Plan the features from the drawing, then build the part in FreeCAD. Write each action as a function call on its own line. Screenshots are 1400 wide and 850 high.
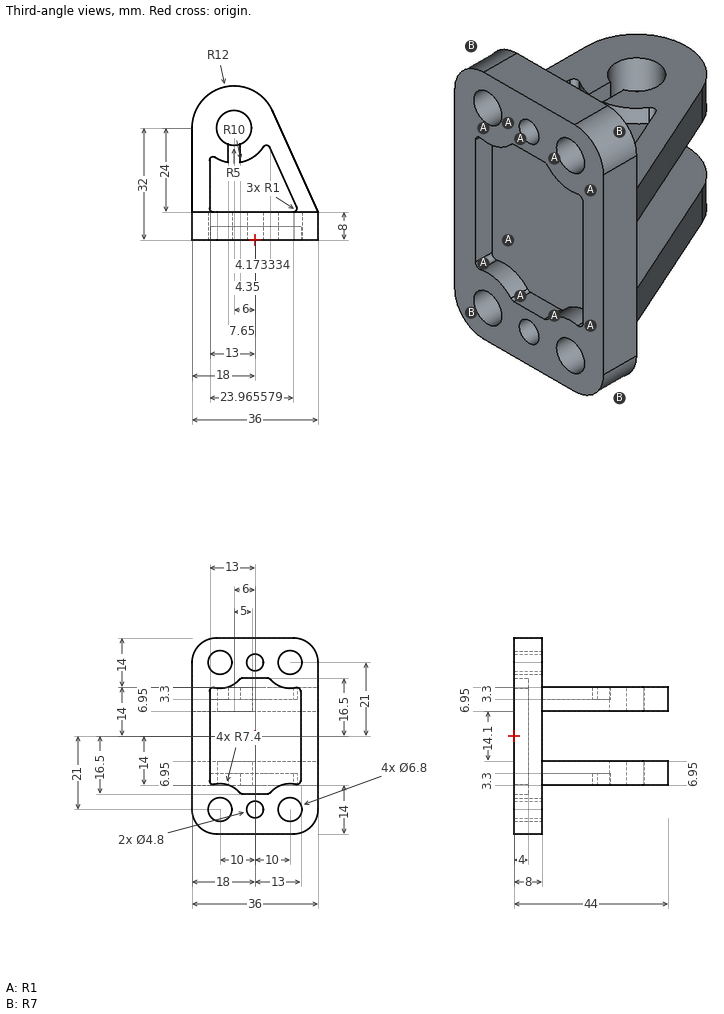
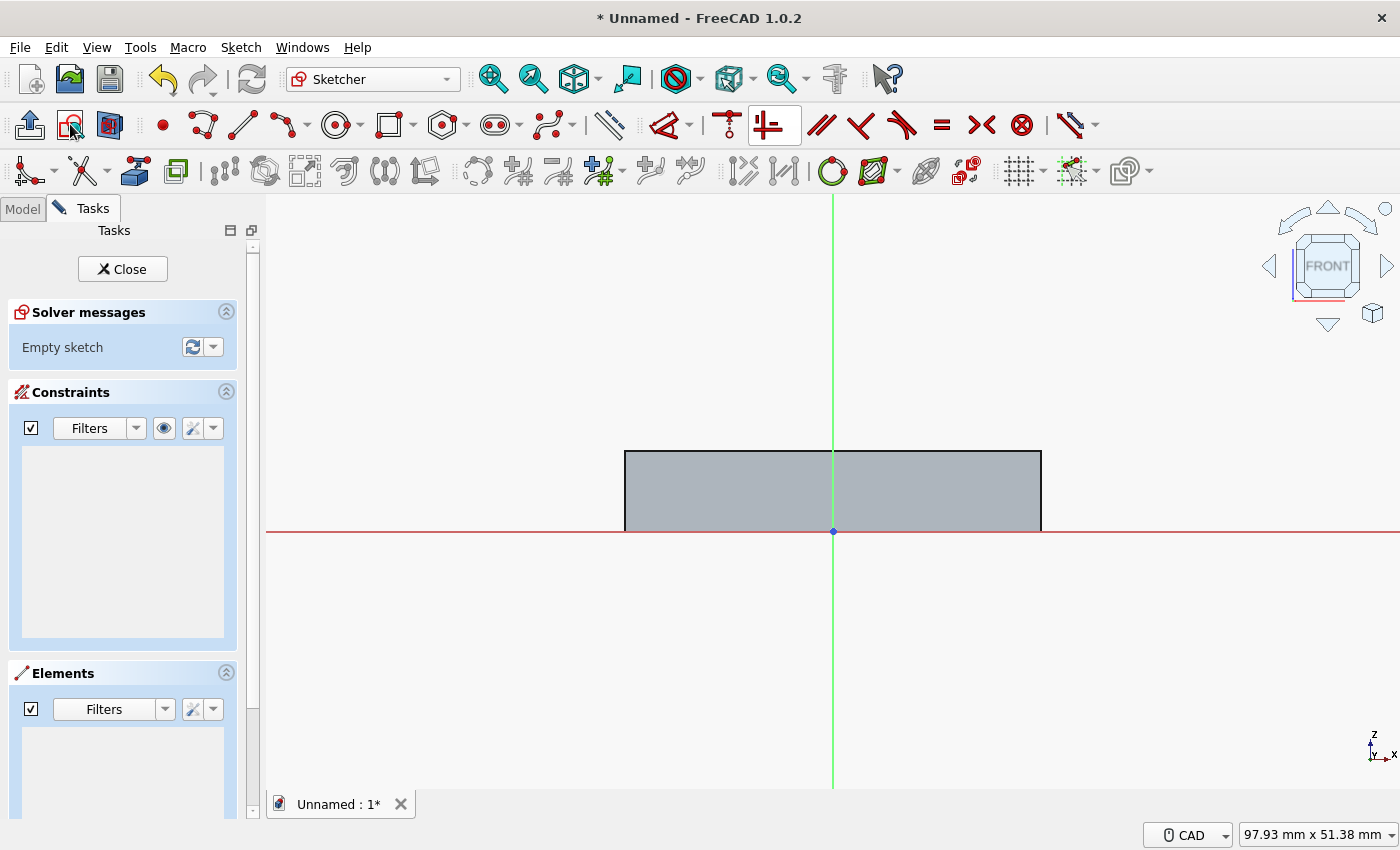
scroll(972, 492, up, 2)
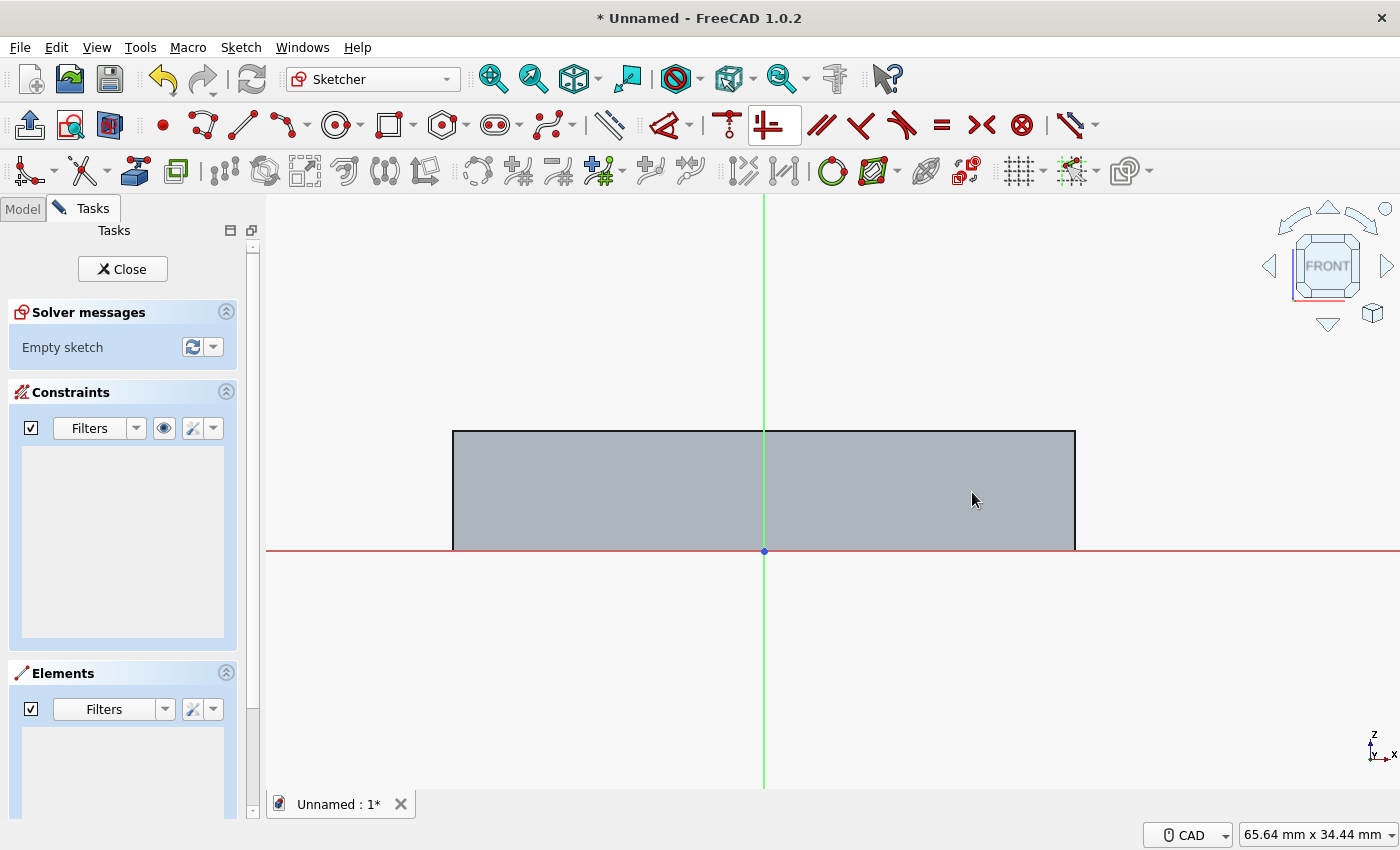
key(g)
key(r)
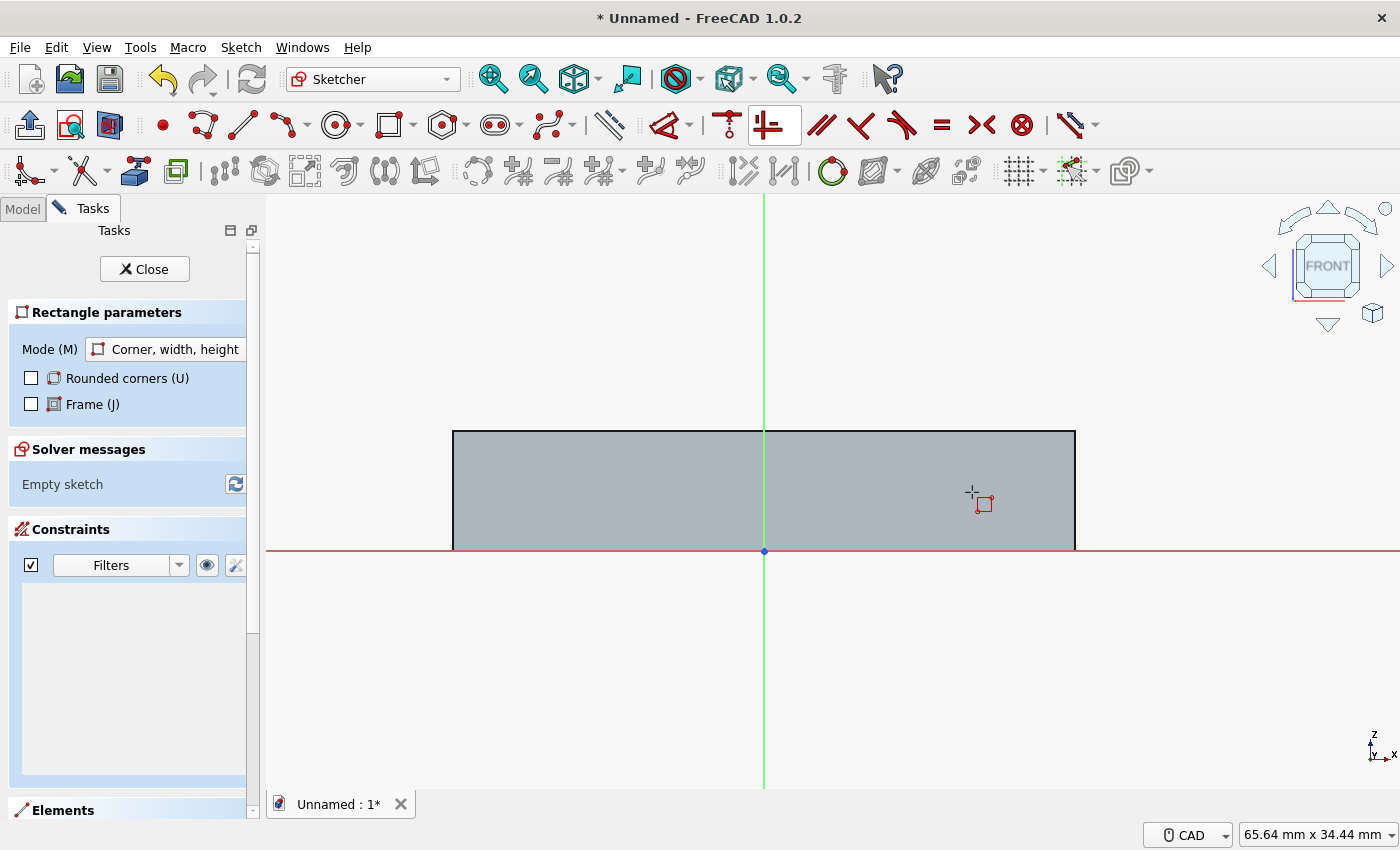
click(453, 431)
click(1075, 551)
key(Escape)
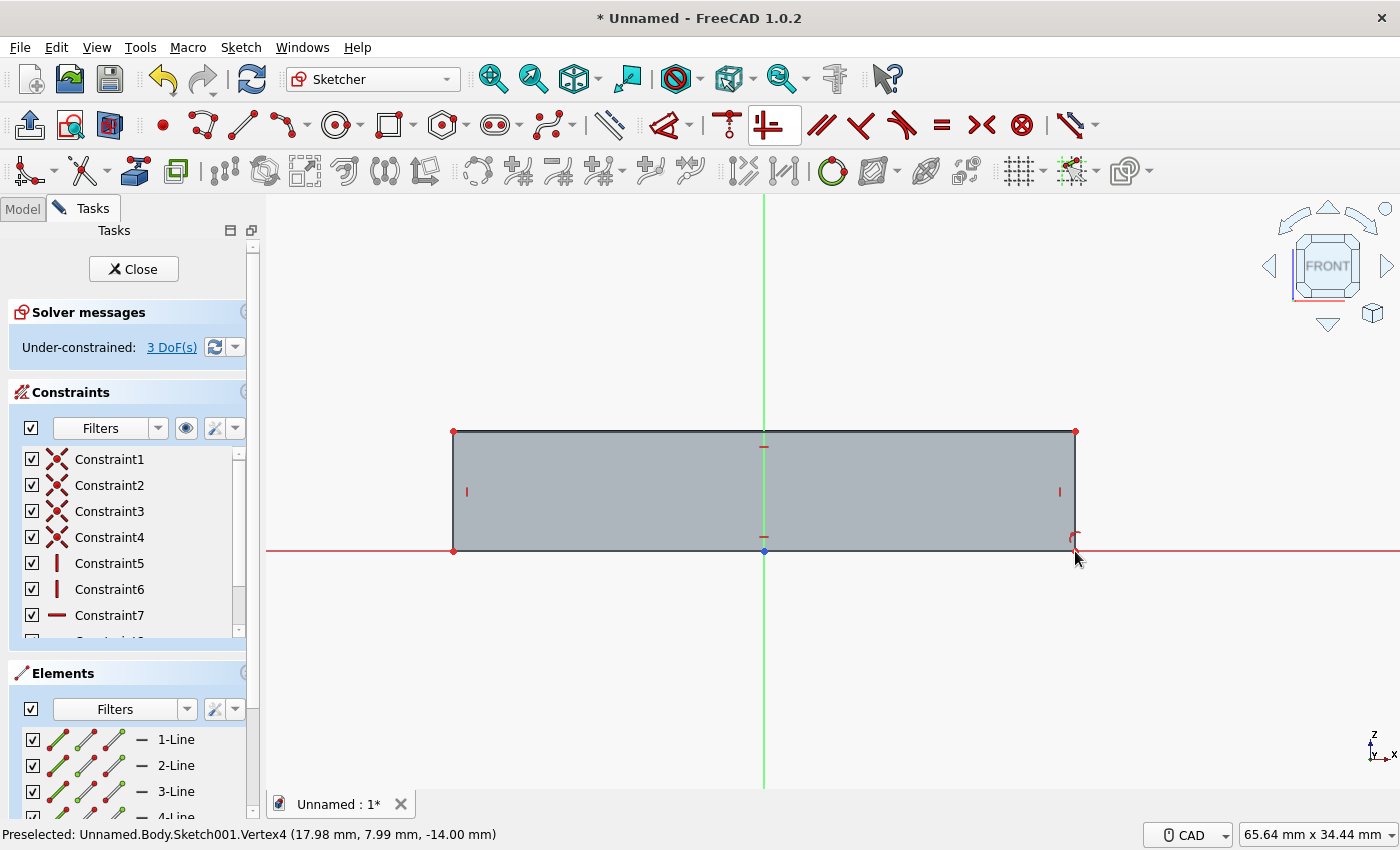
click(640, 551)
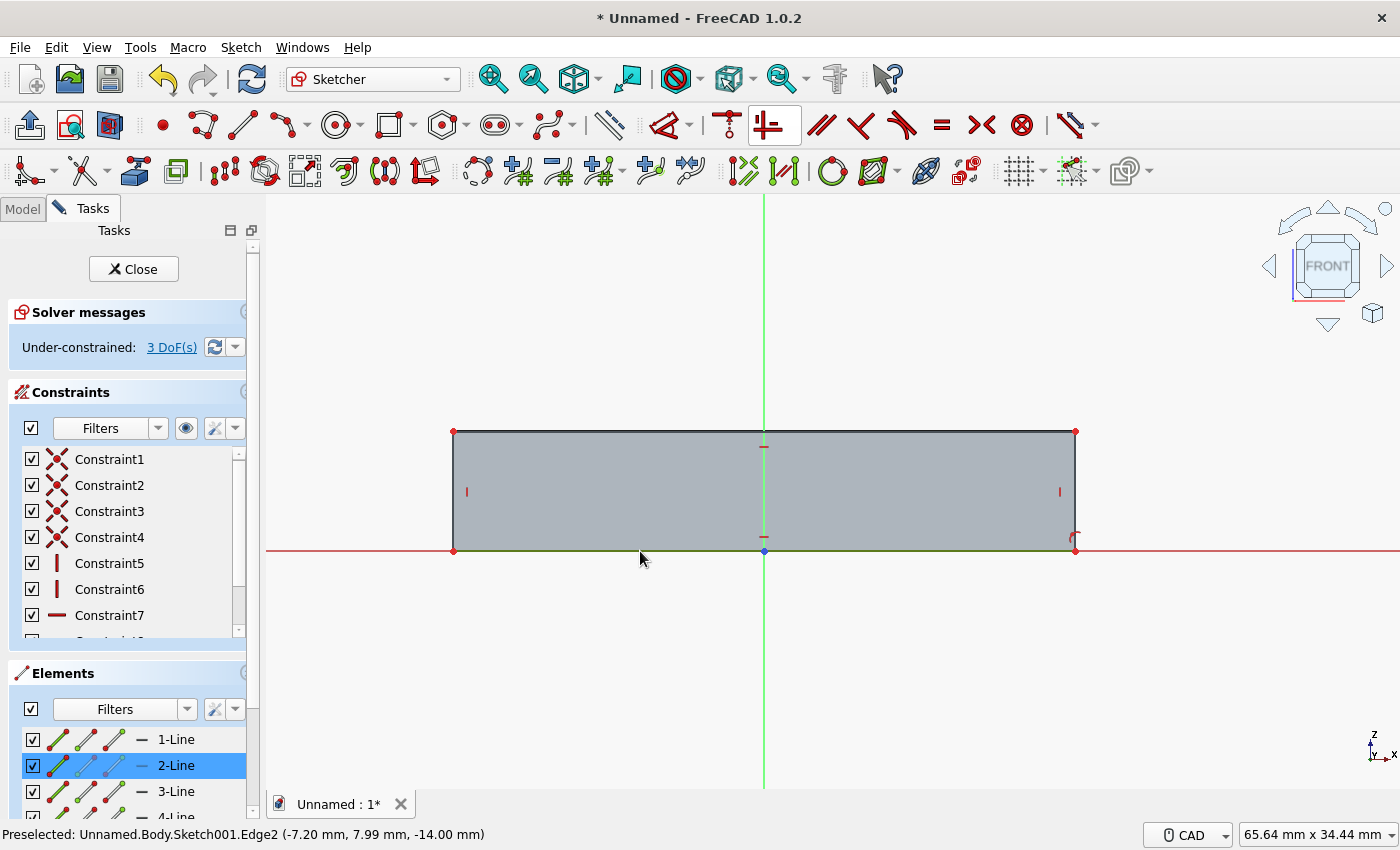
key(l)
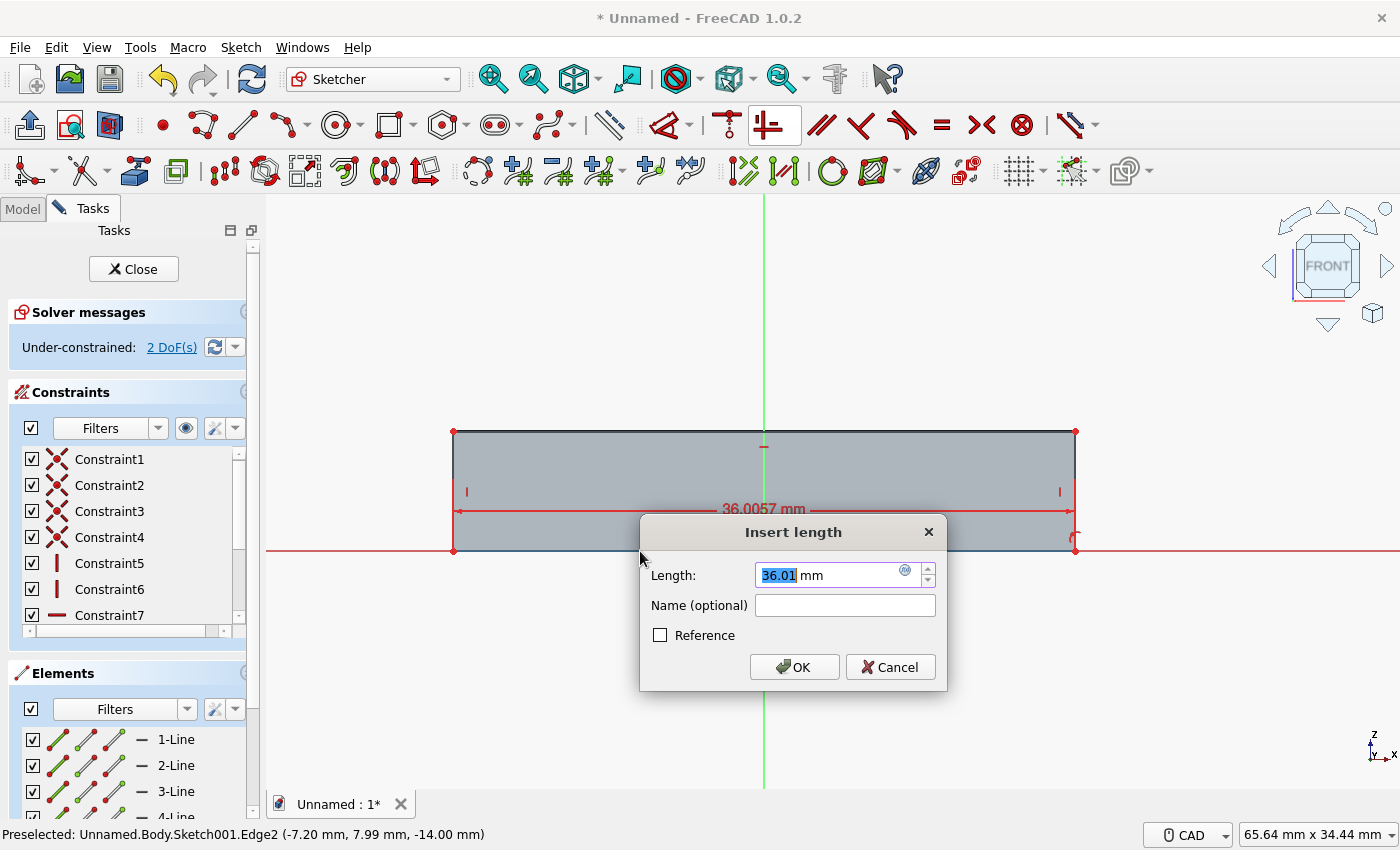
text(36)
key(Return)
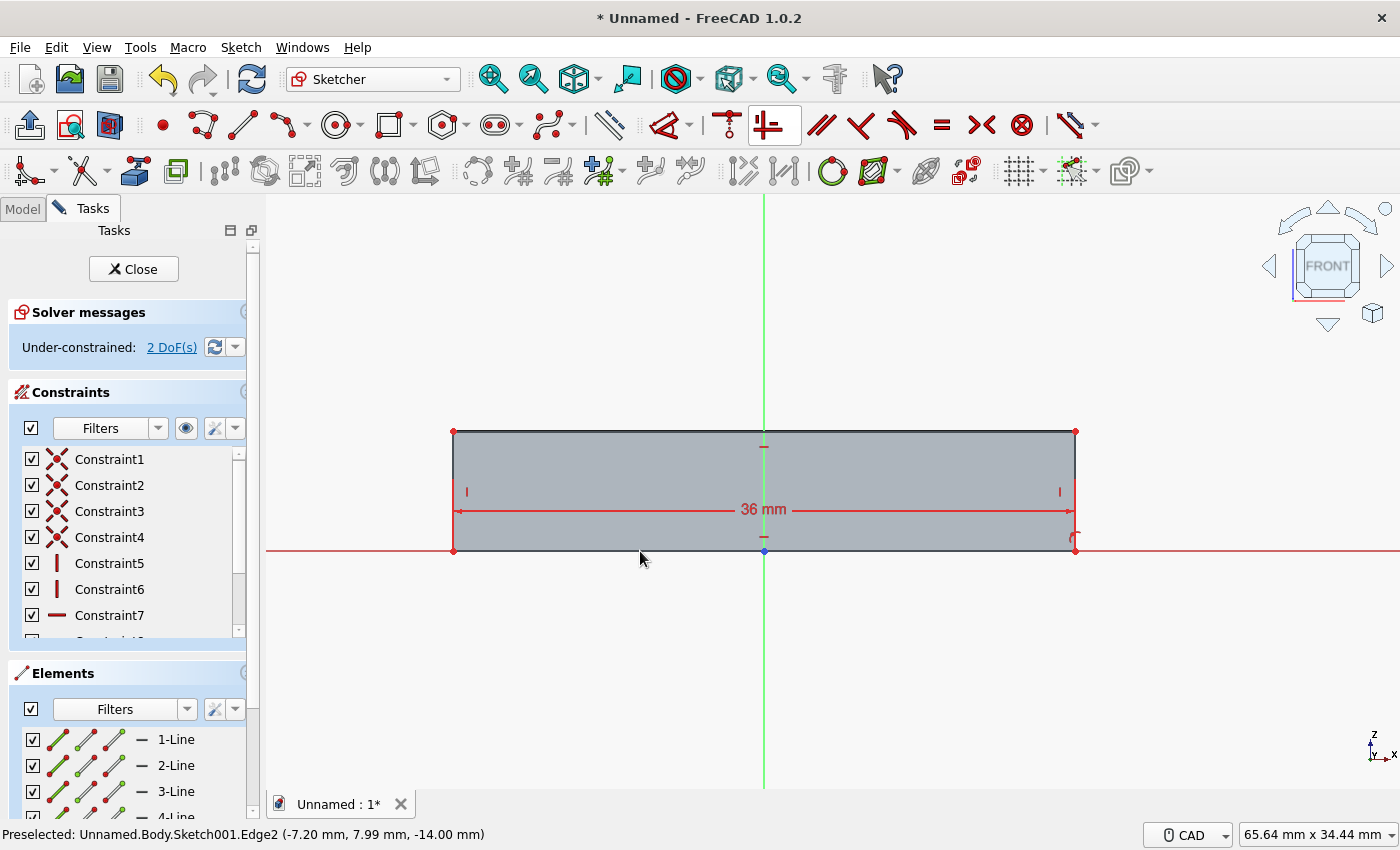
click(453, 432)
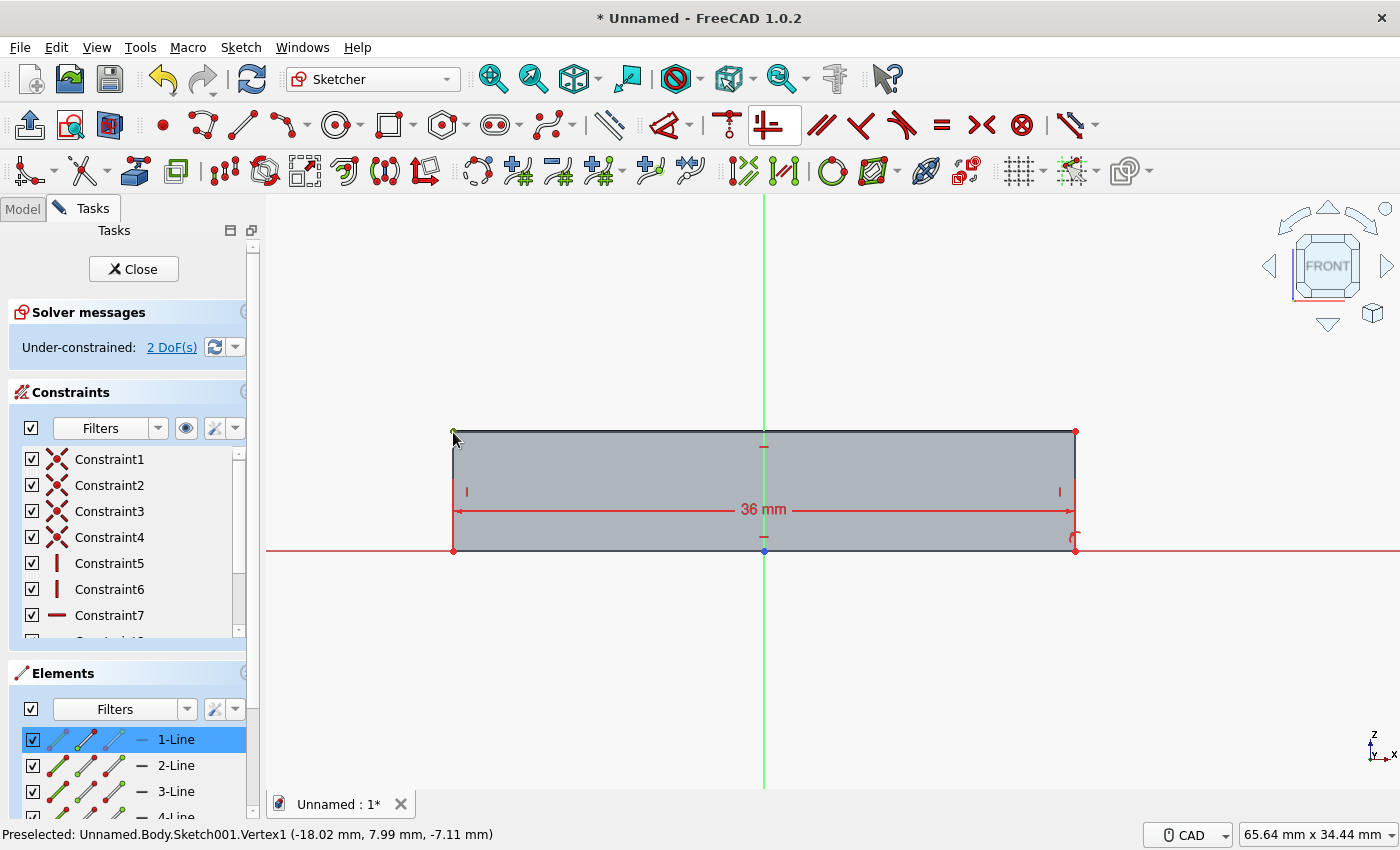
key(l)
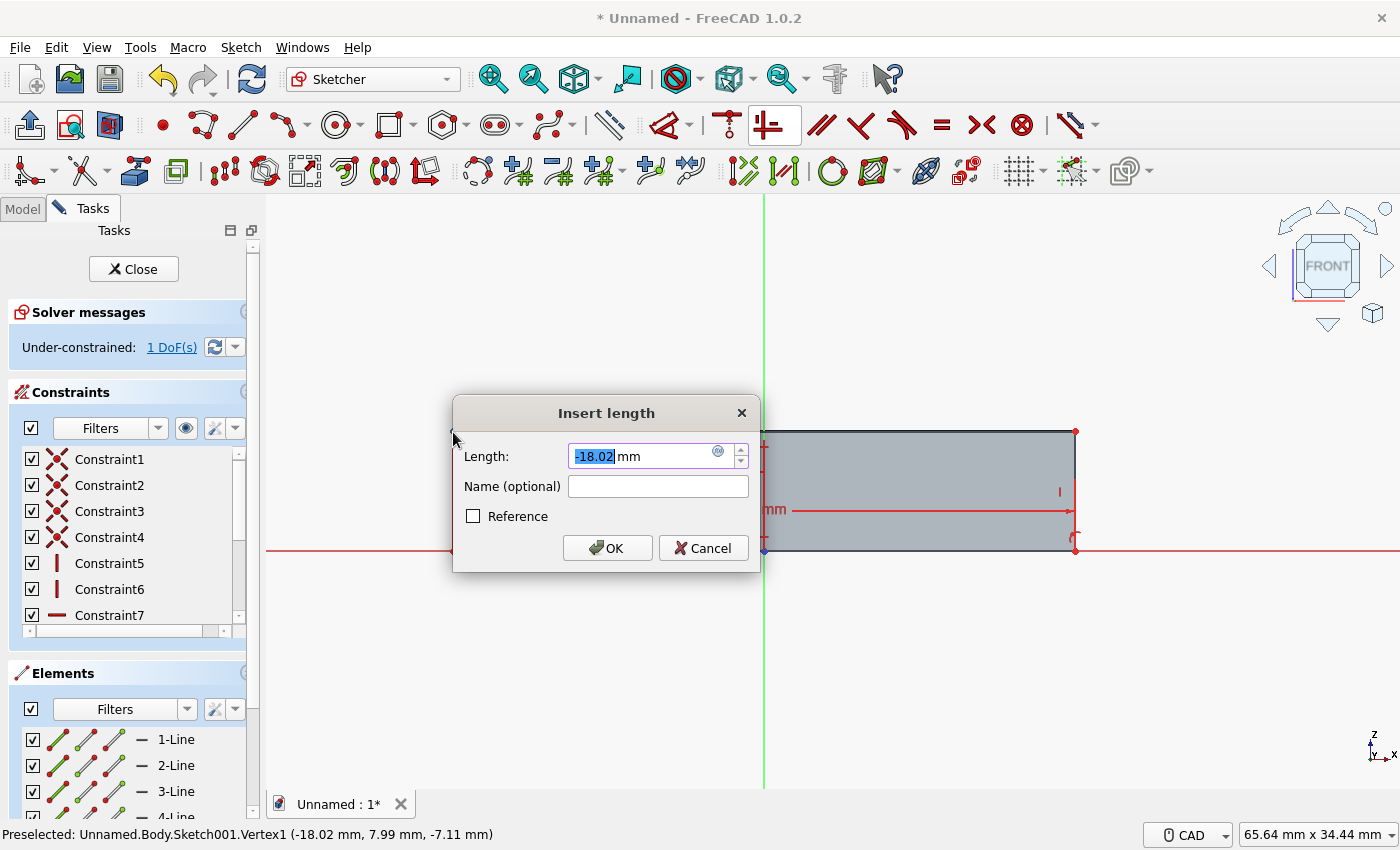
text(-18)
key(Return)